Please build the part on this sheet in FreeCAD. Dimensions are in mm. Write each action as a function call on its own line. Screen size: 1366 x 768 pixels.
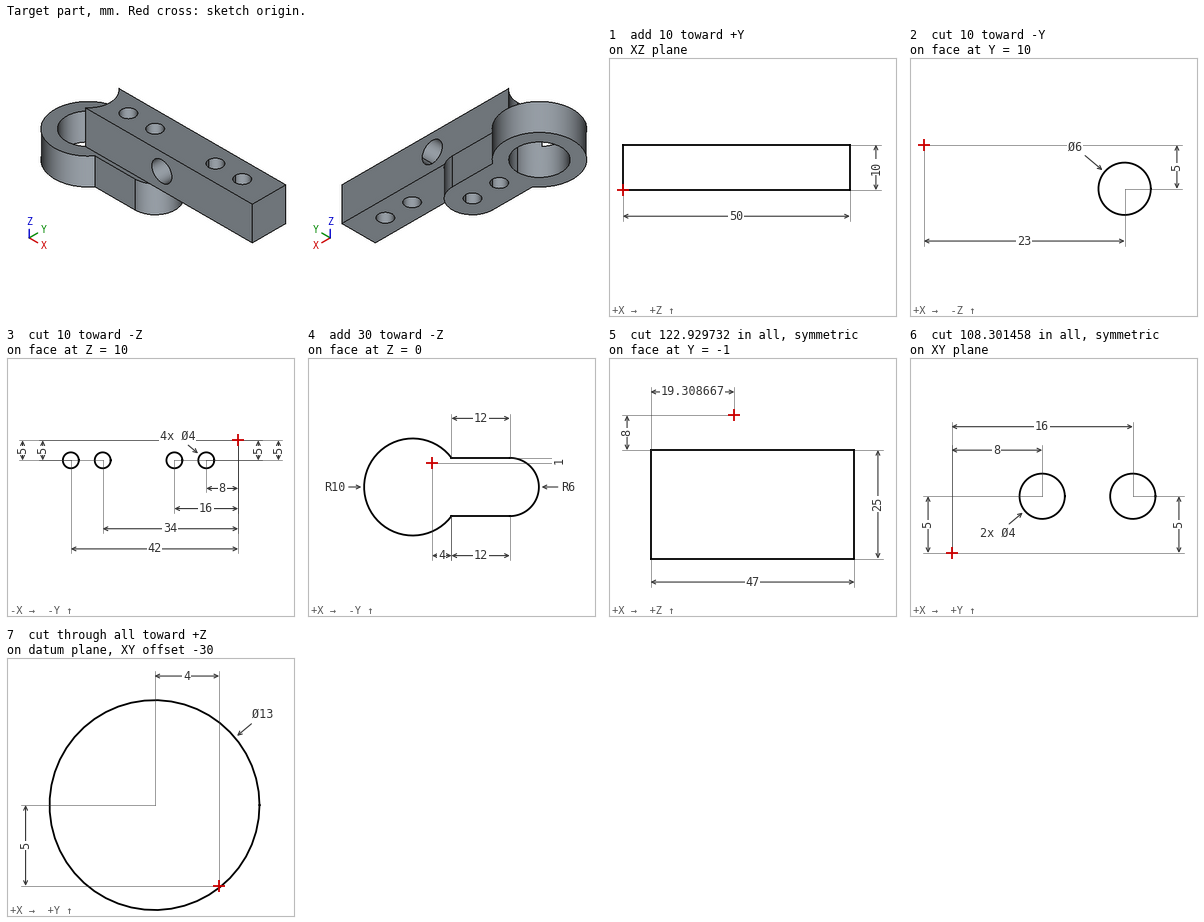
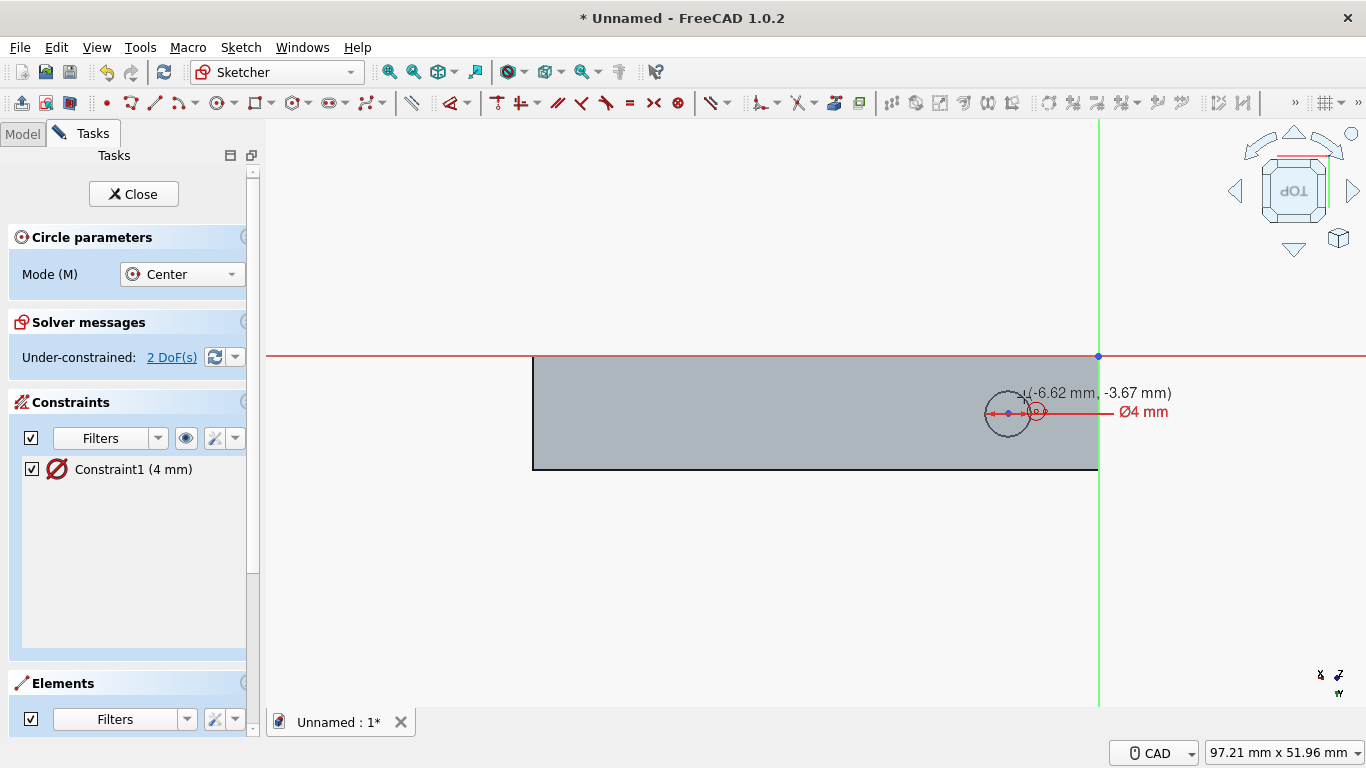
click(918, 413)
move(934, 397)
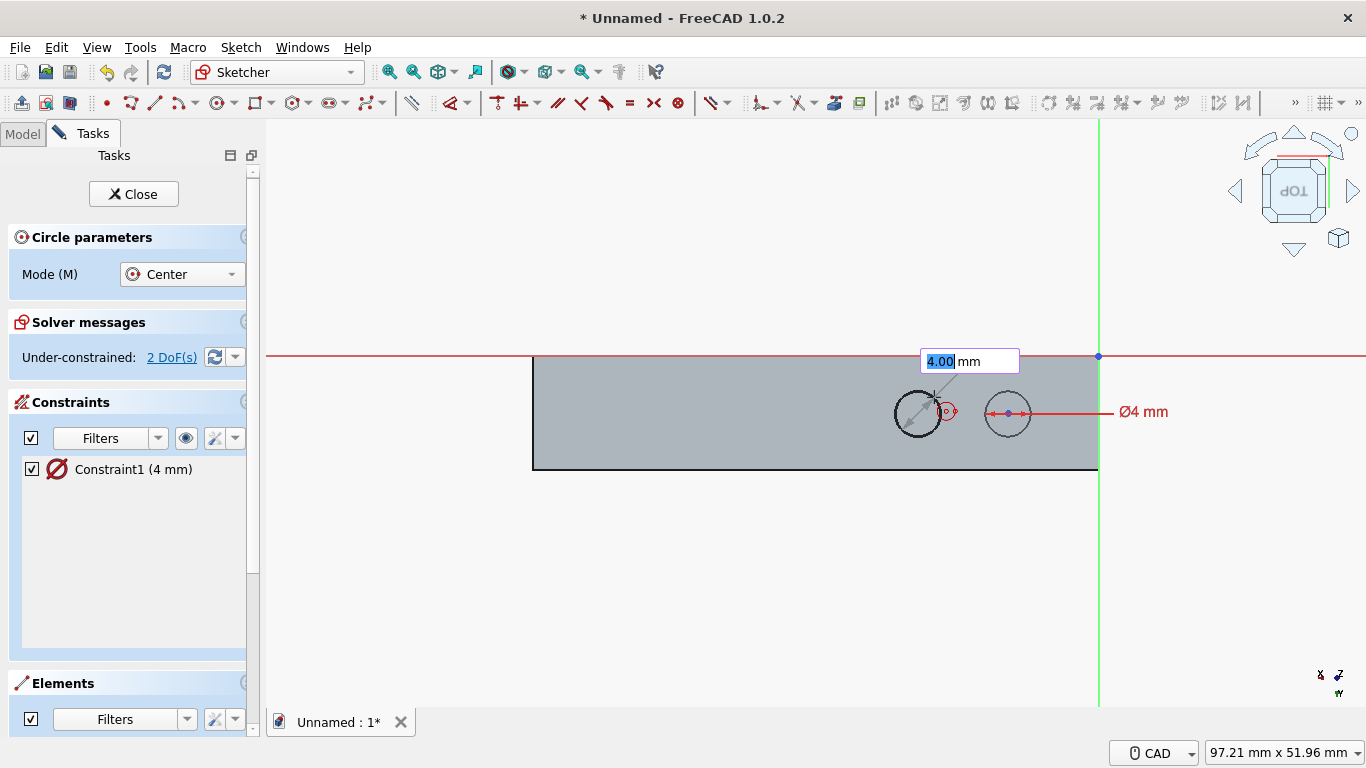
text(4)
key(Return)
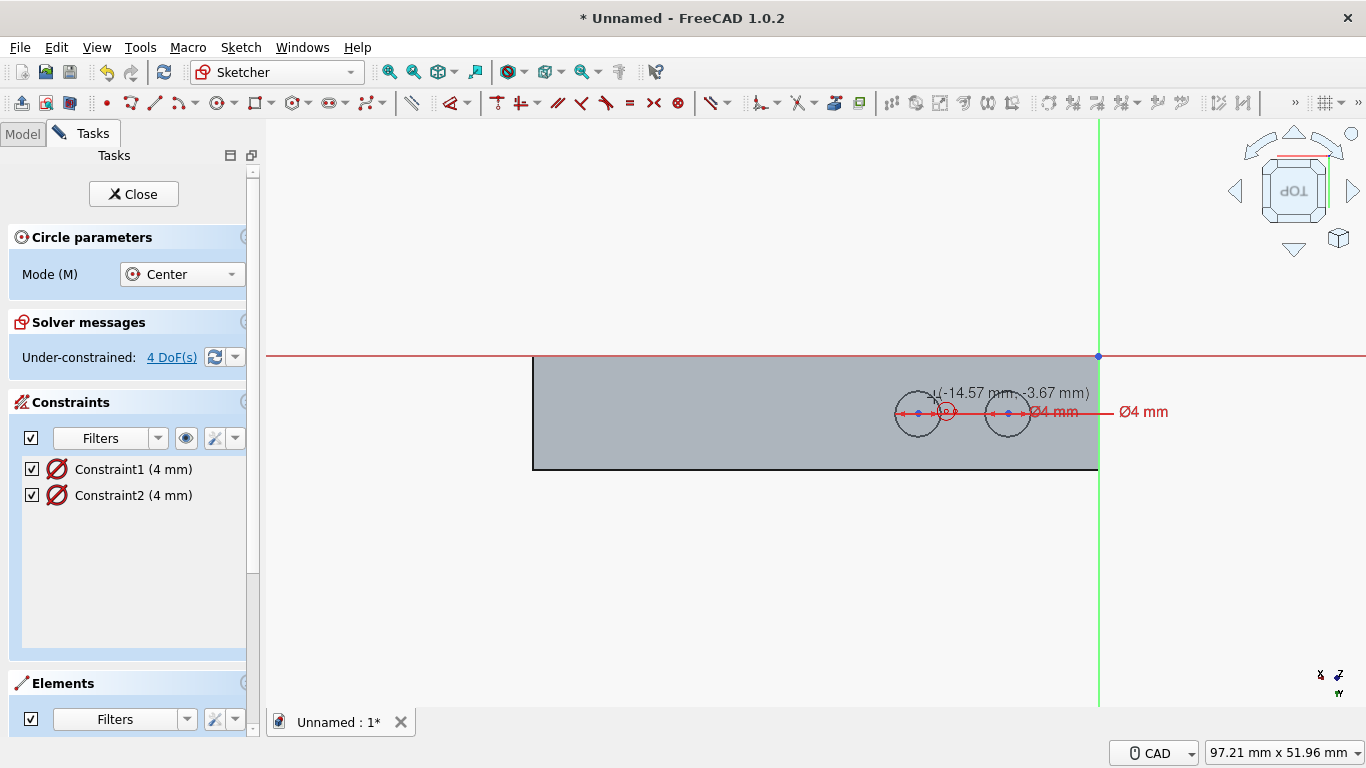
click(624, 413)
move(640, 397)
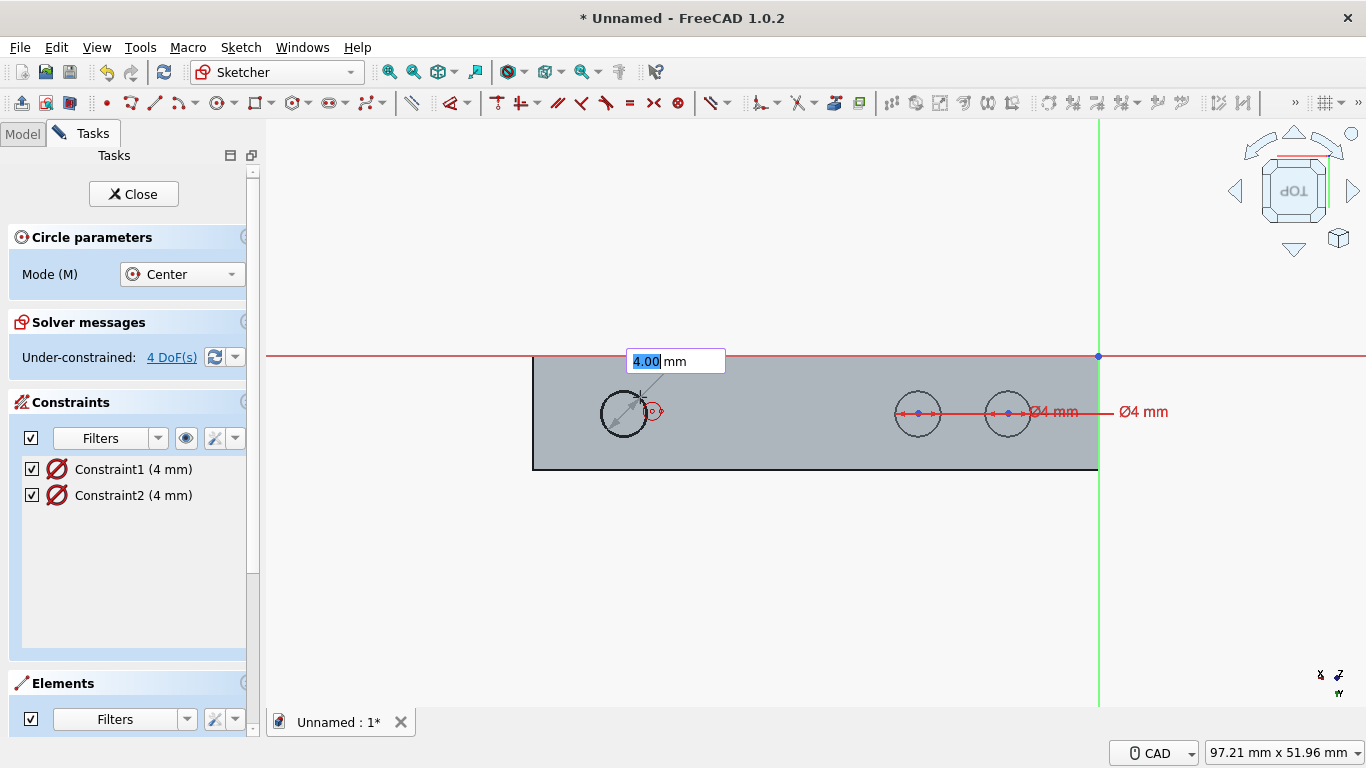
text(4)
key(Return)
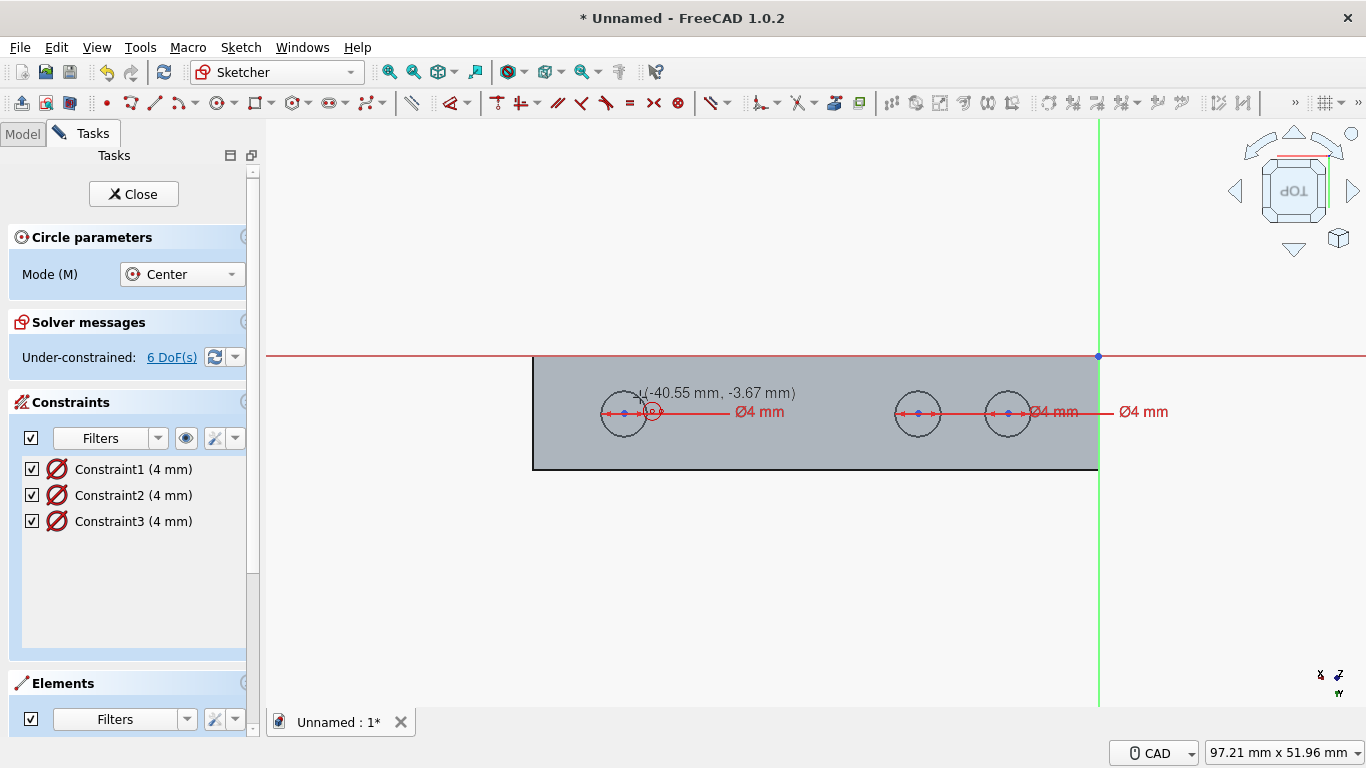
click(714, 413)
move(730, 397)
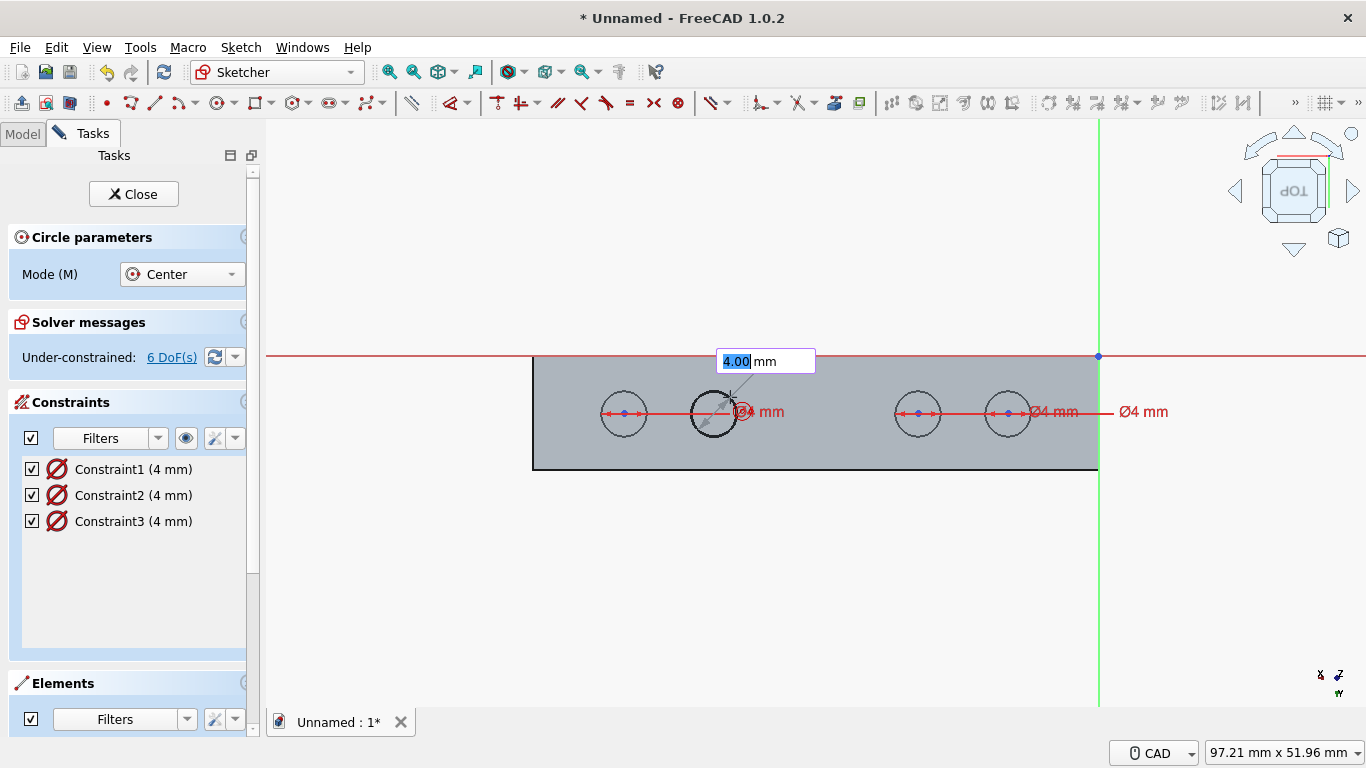
text(4)
key(Return)
key(Escape)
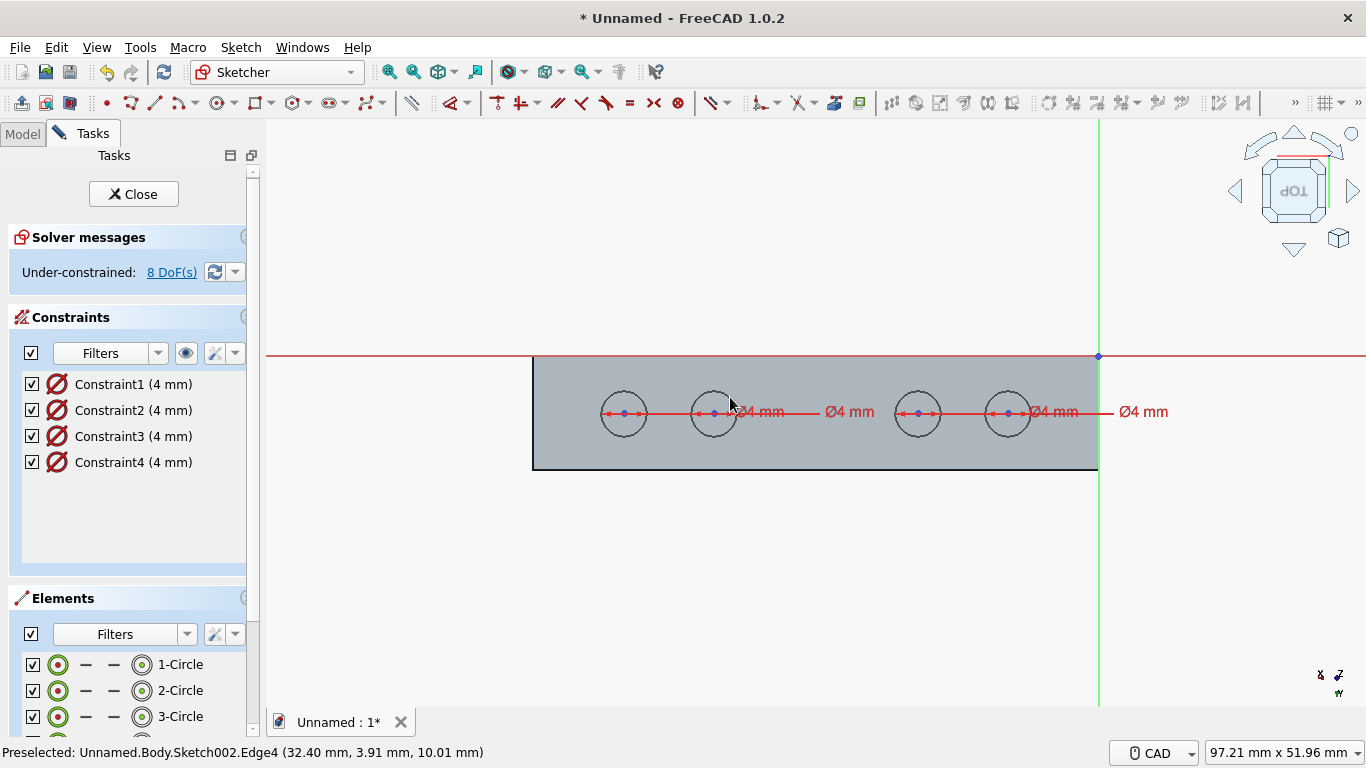
click(450, 104)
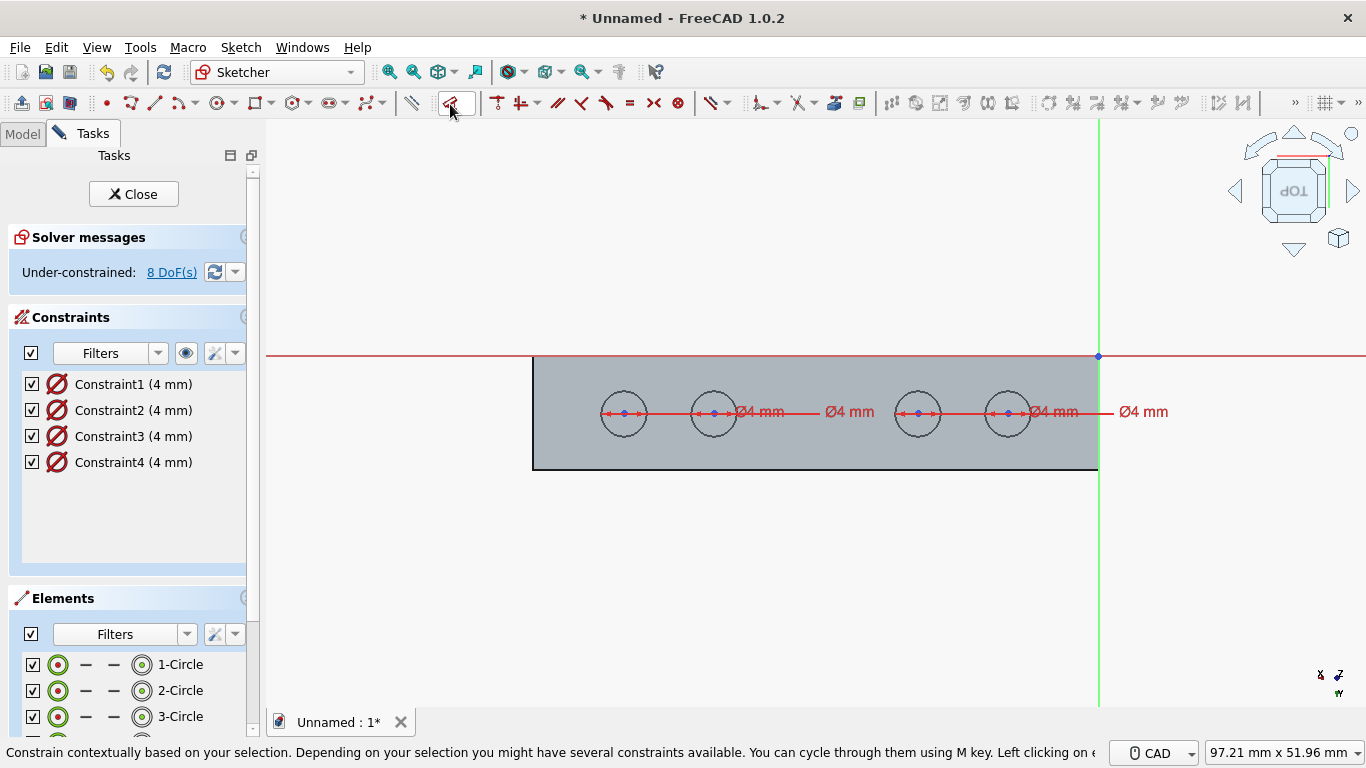
click(1008, 414)
click(1053, 322)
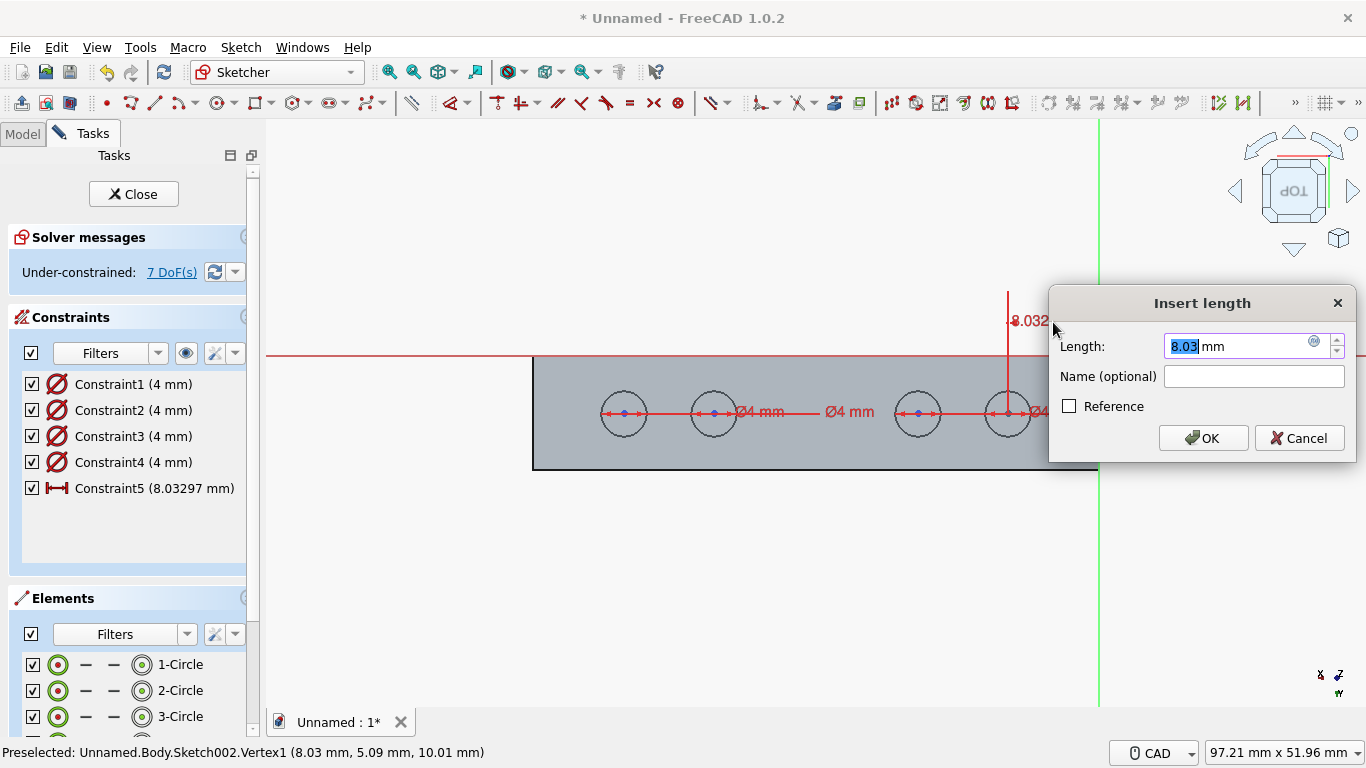
text(8)
key(Return)